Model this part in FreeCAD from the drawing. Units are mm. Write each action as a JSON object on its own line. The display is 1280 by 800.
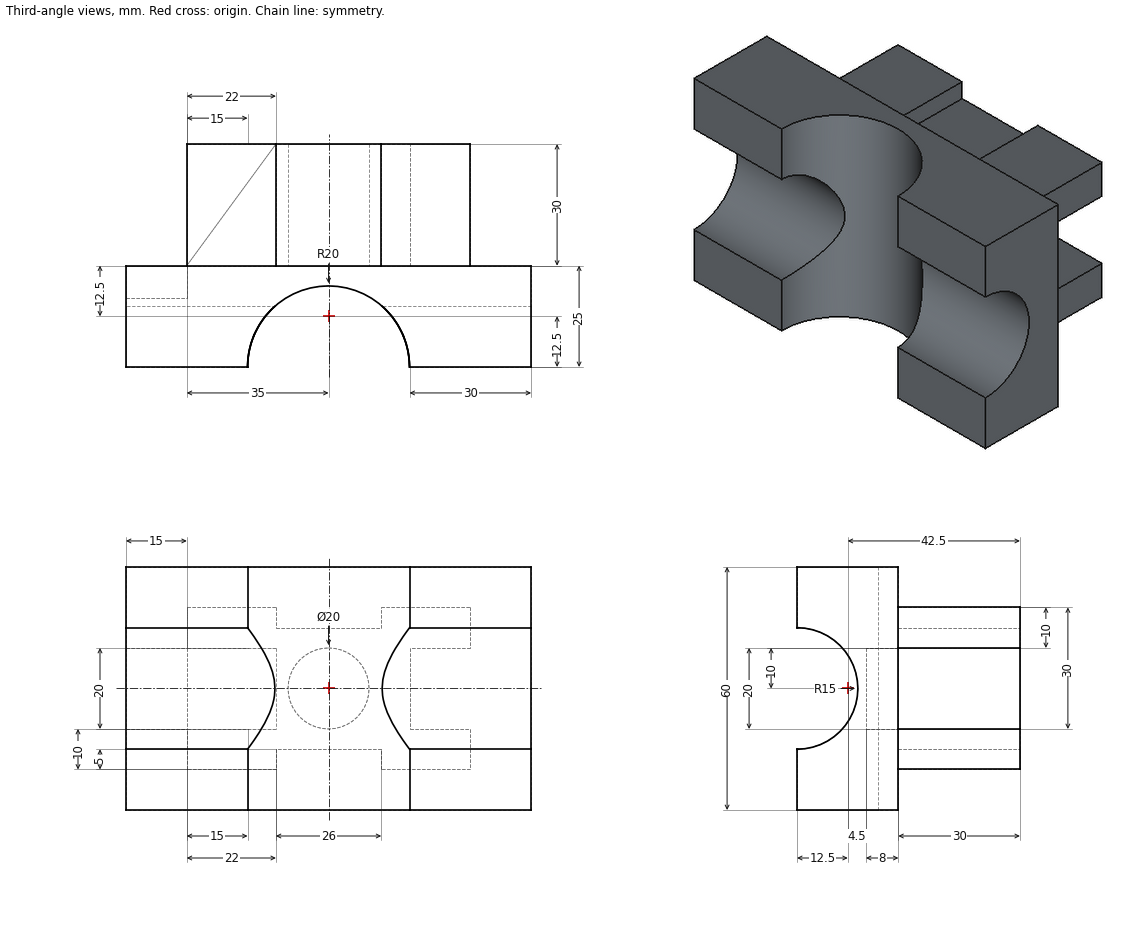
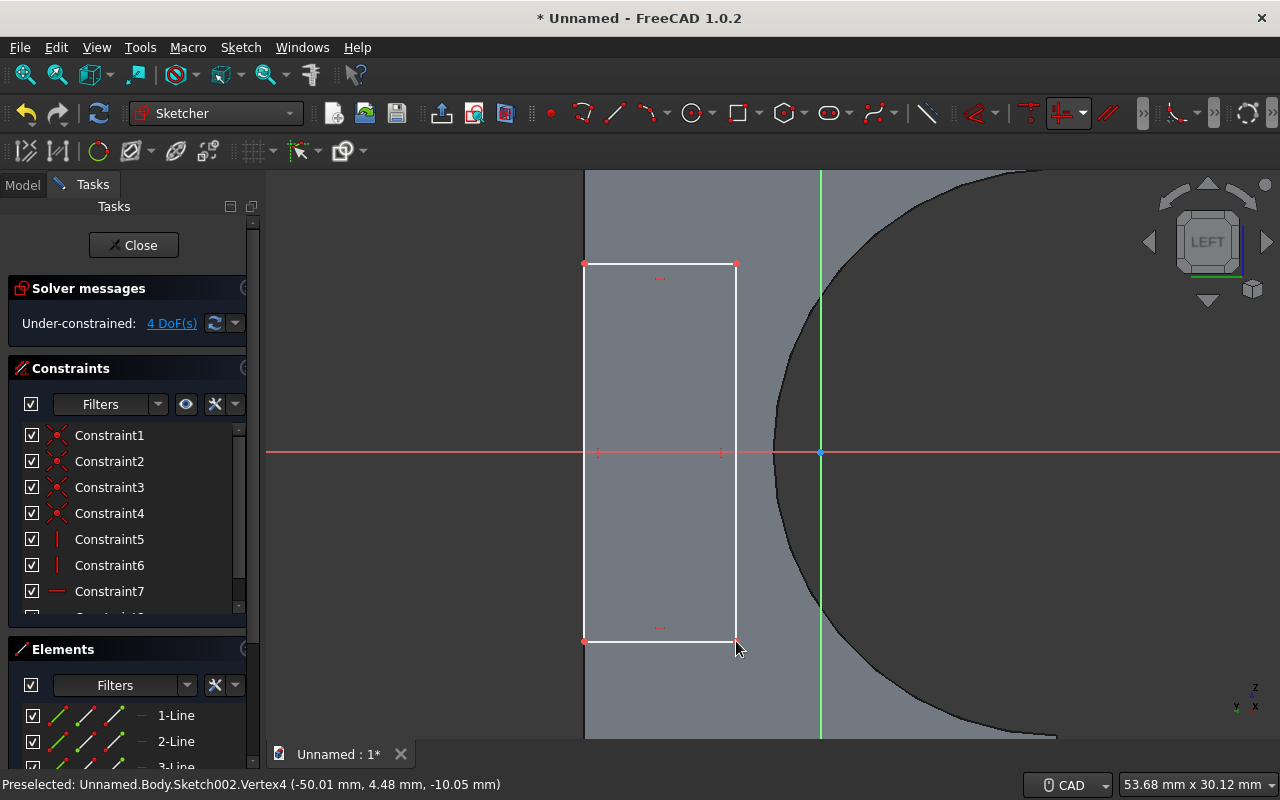
{"action": "key", "text": "d"}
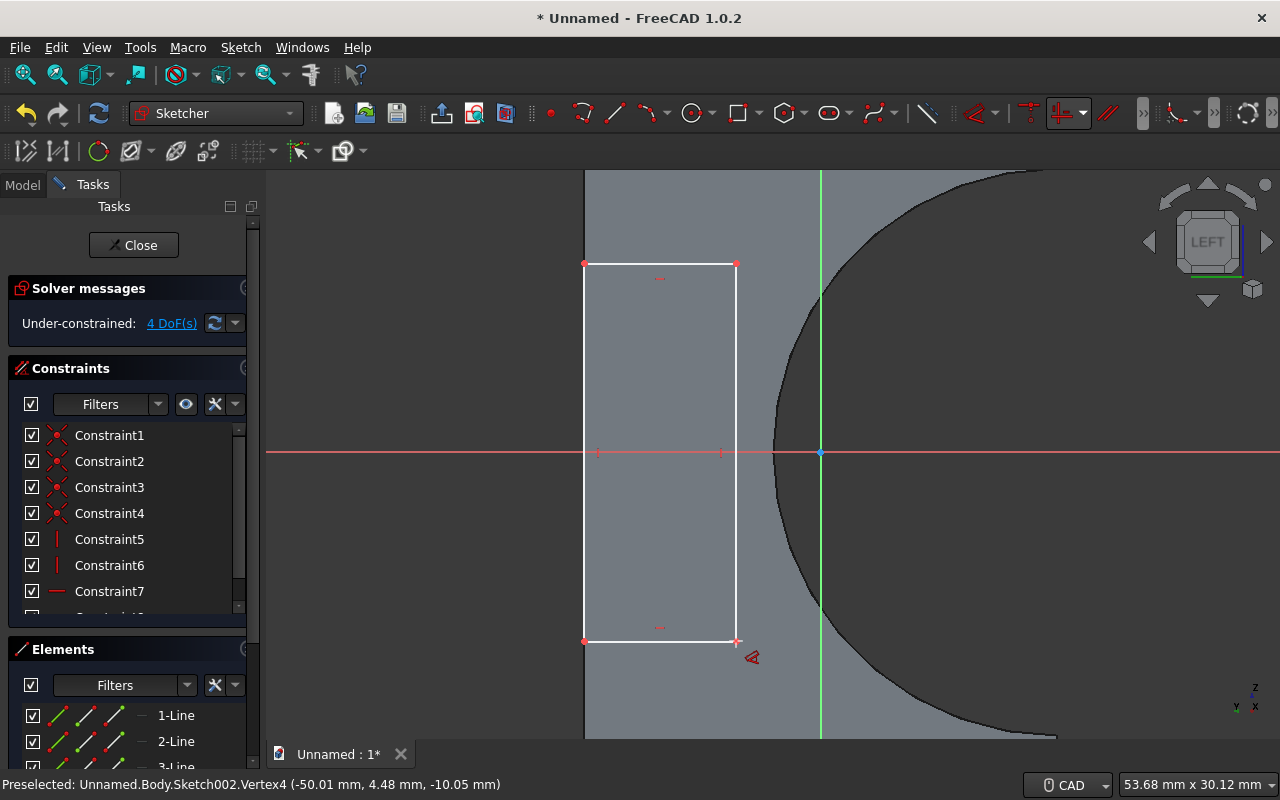
{"action": "left_click", "coordinate": [630, 642]}
{"action": "left_click", "coordinate": [660, 676]}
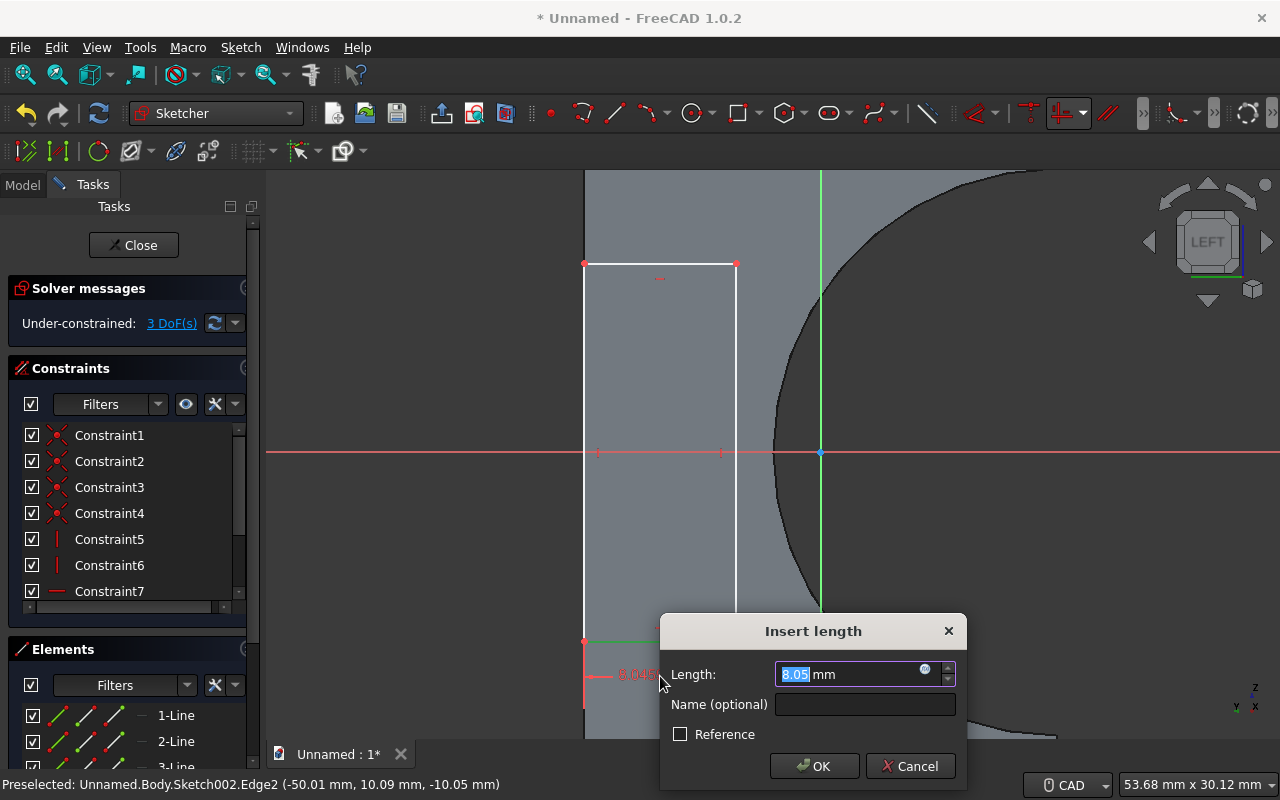
{"action": "type", "text": "8"}
{"action": "key", "text": "Return"}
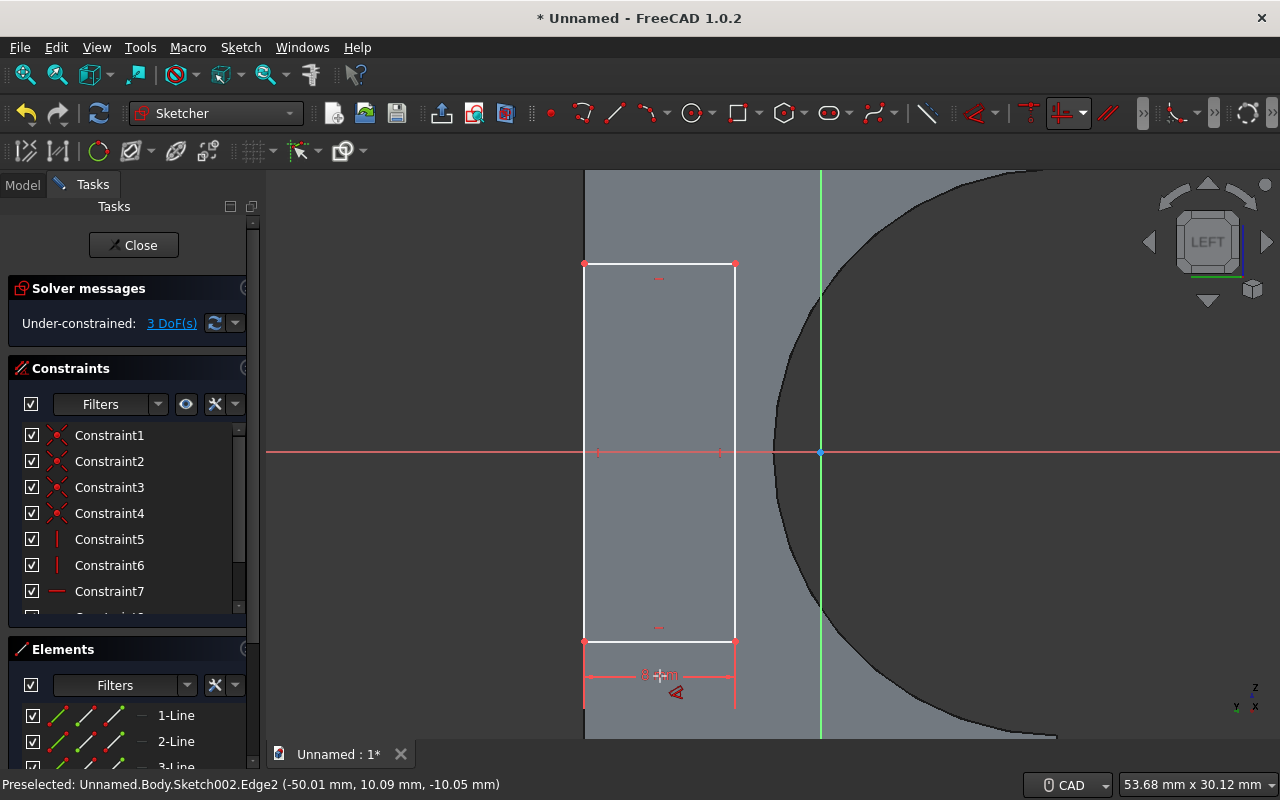
{"action": "left_click", "coordinate": [584, 377]}
{"action": "left_click", "coordinate": [550, 366]}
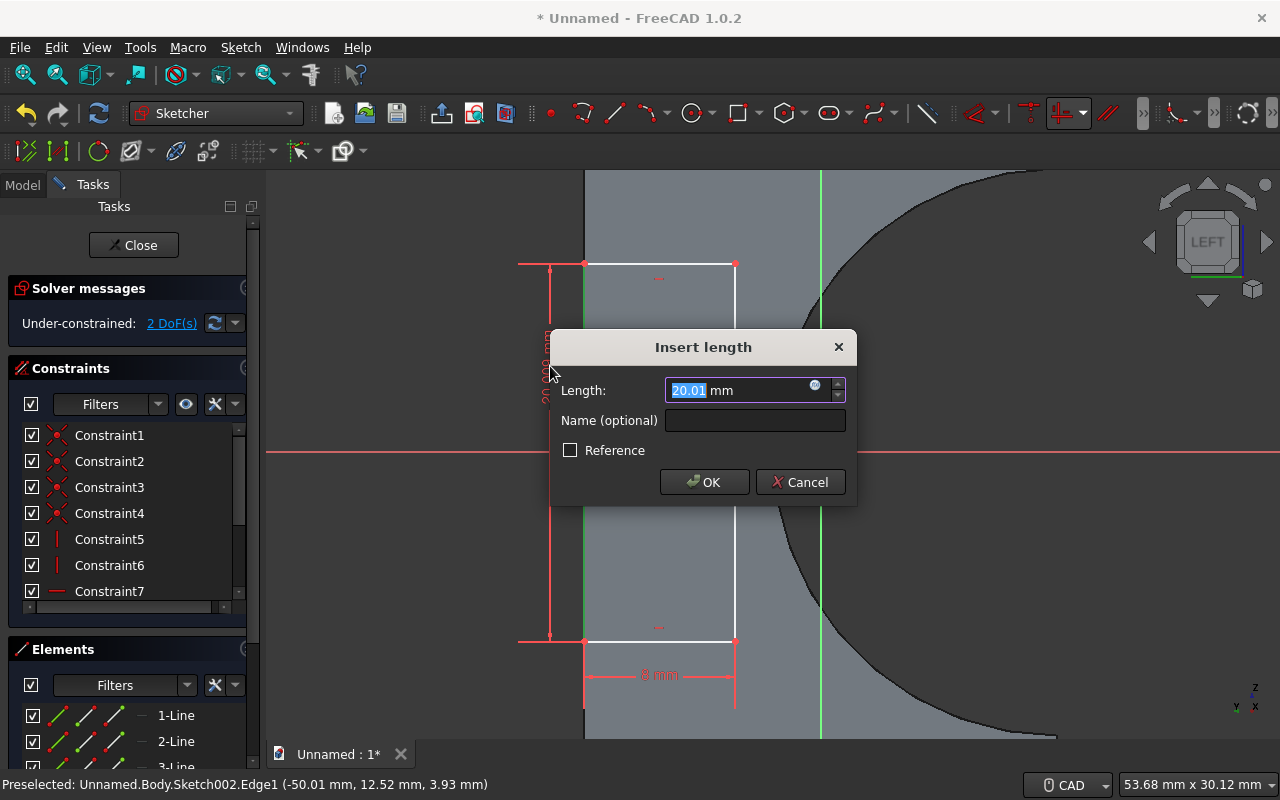
{"action": "type", "text": "20"}
{"action": "key", "text": "Return"}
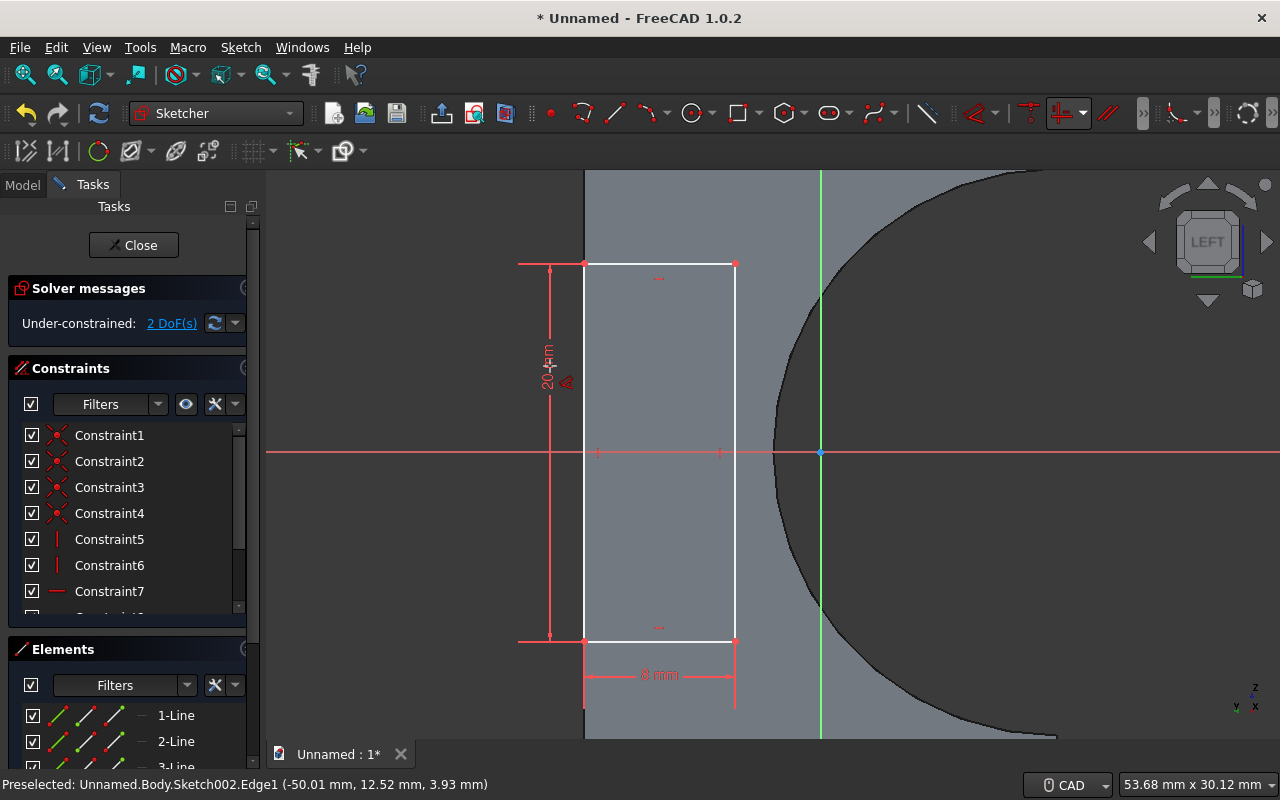
{"action": "left_click", "coordinate": [584, 264]}
{"action": "left_click", "coordinate": [550, 315]}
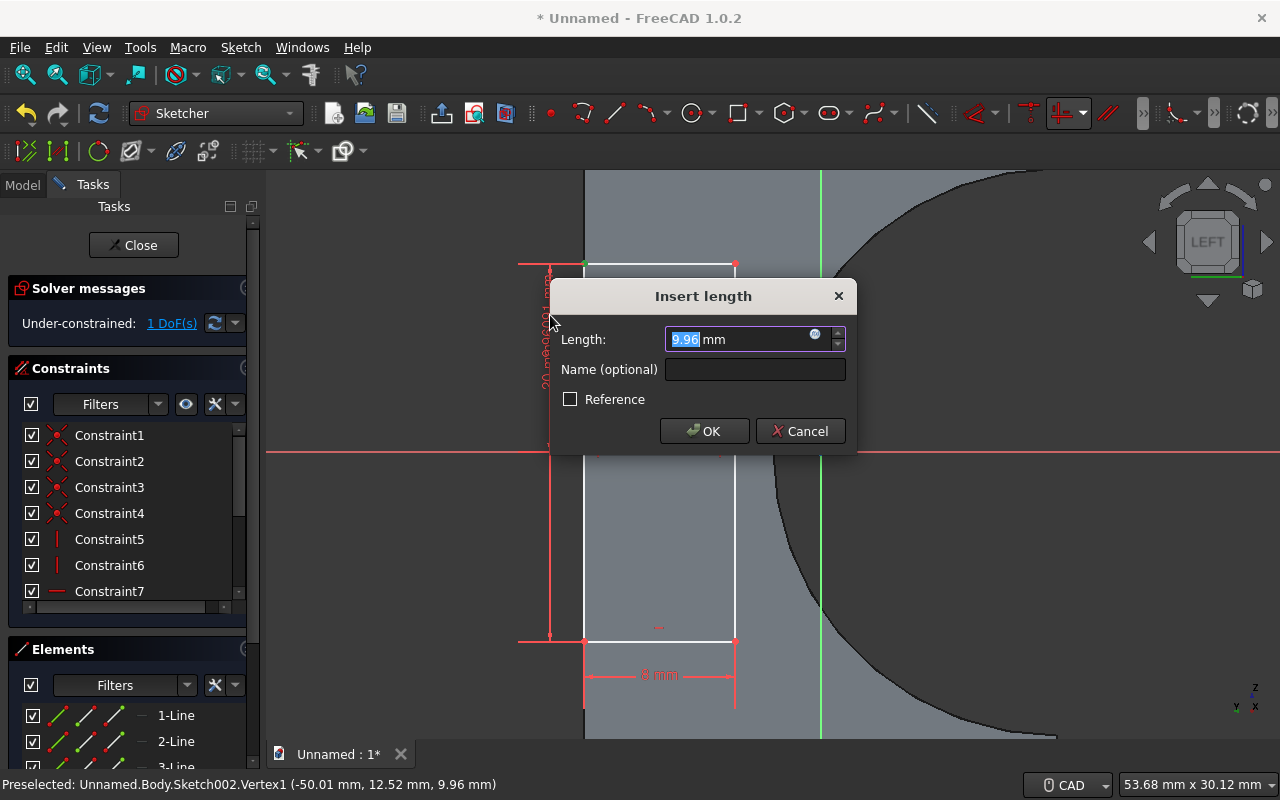
{"action": "type", "text": "10"}
{"action": "key", "text": "Return"}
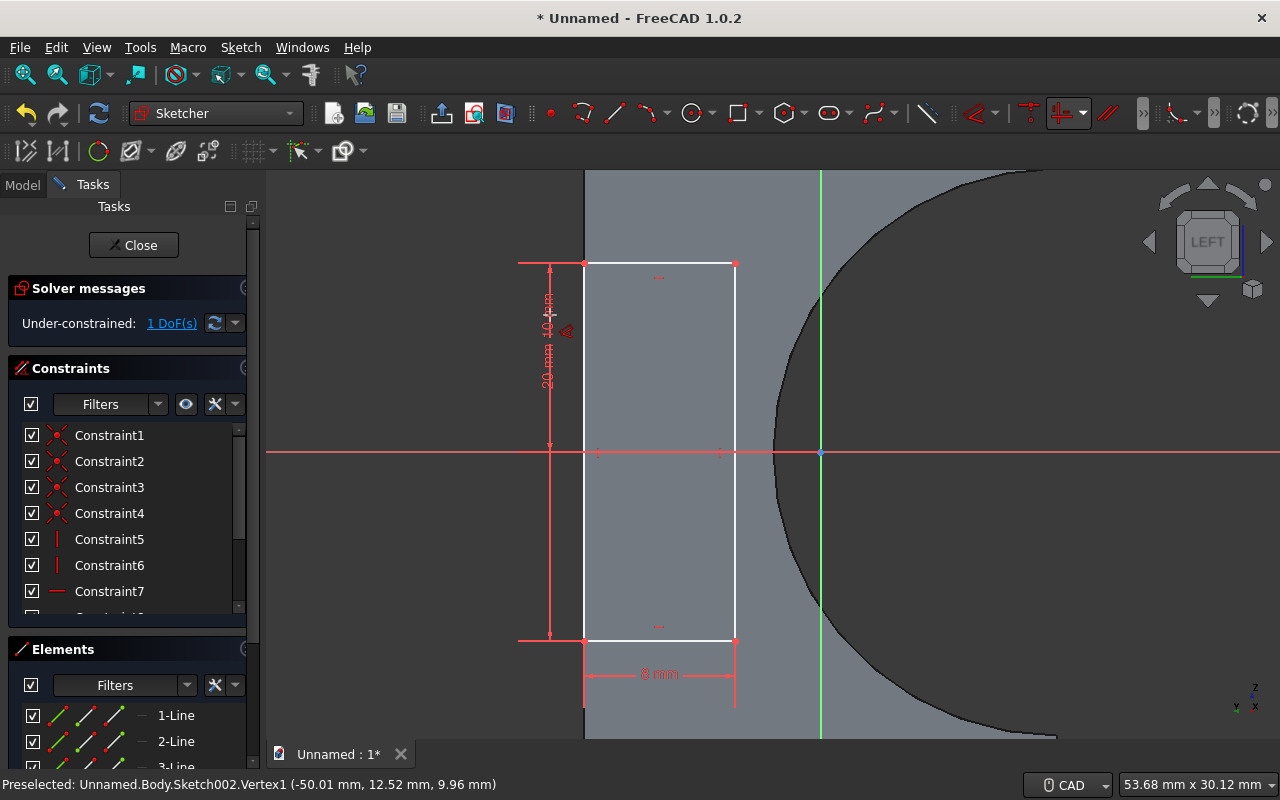
{"action": "left_click", "coordinate": [735, 641]}
{"action": "left_click", "coordinate": [778, 675]}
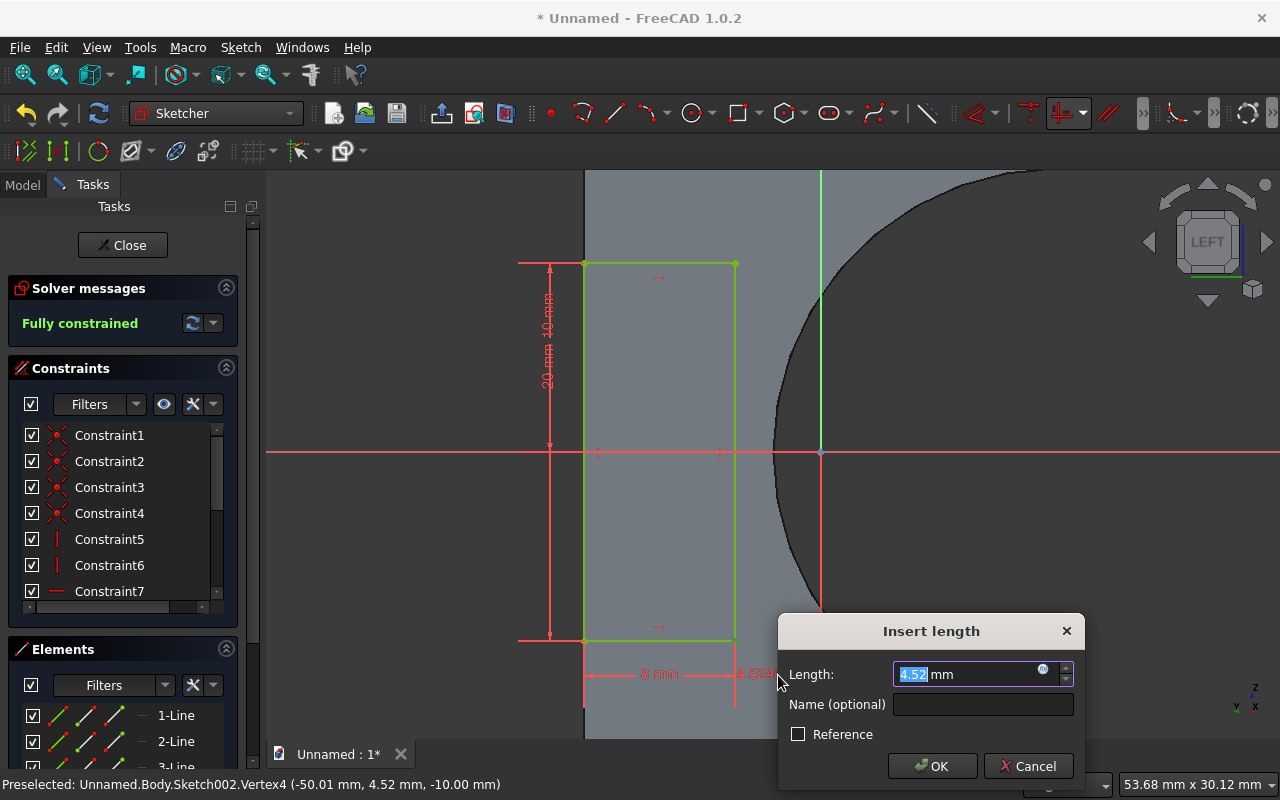
{"action": "type", "text": "4.5"}
{"action": "key", "text": "Return"}
{"action": "key", "text": "Escape"}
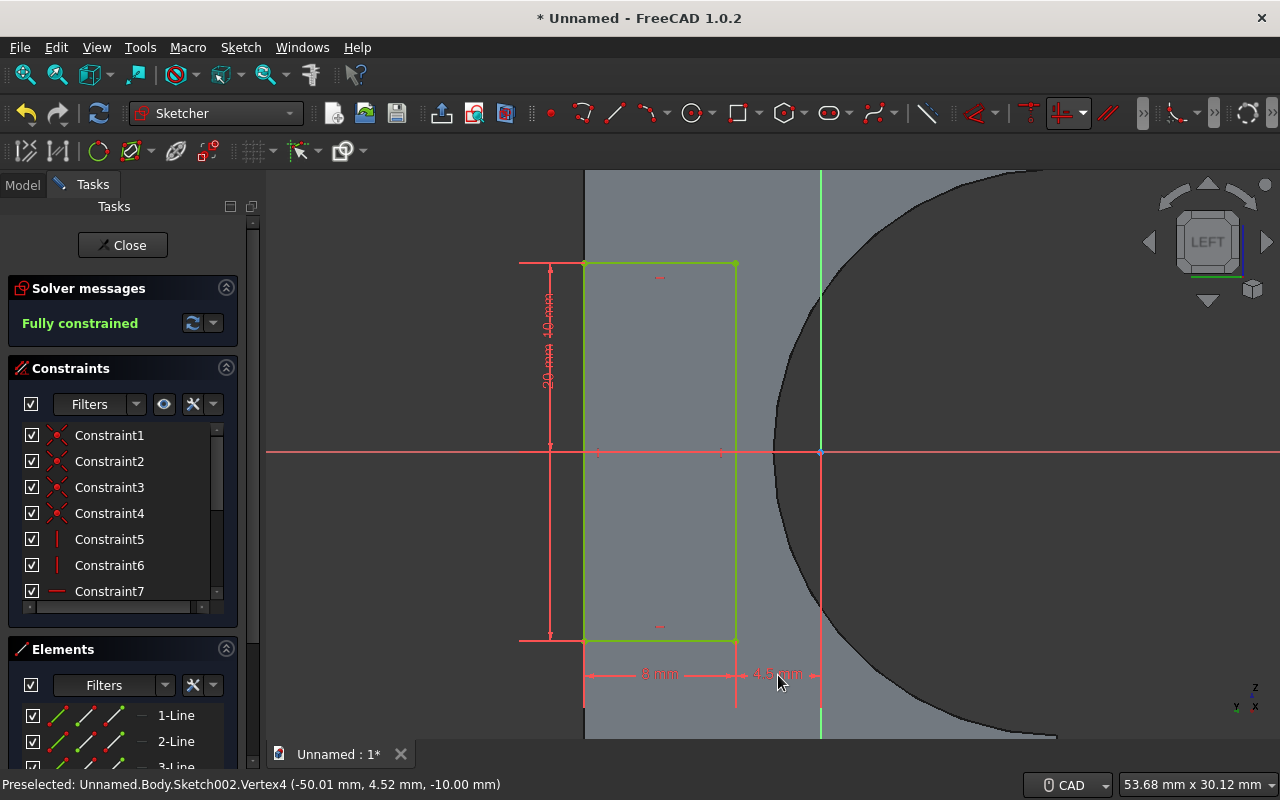
{"action": "left_click", "coordinate": [123, 245]}